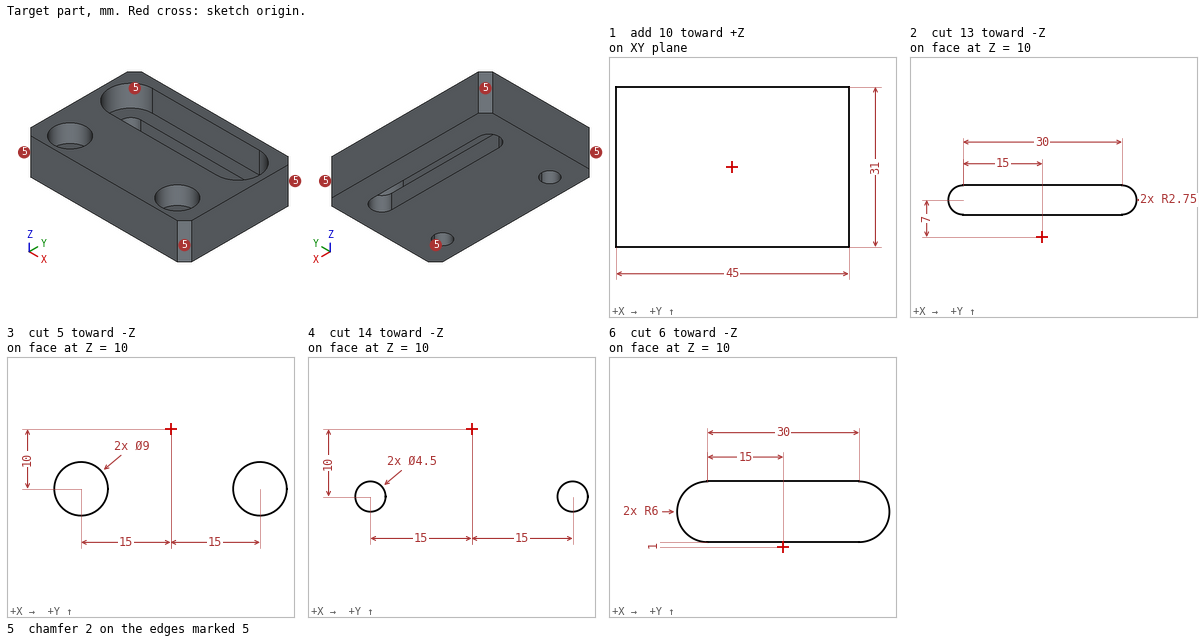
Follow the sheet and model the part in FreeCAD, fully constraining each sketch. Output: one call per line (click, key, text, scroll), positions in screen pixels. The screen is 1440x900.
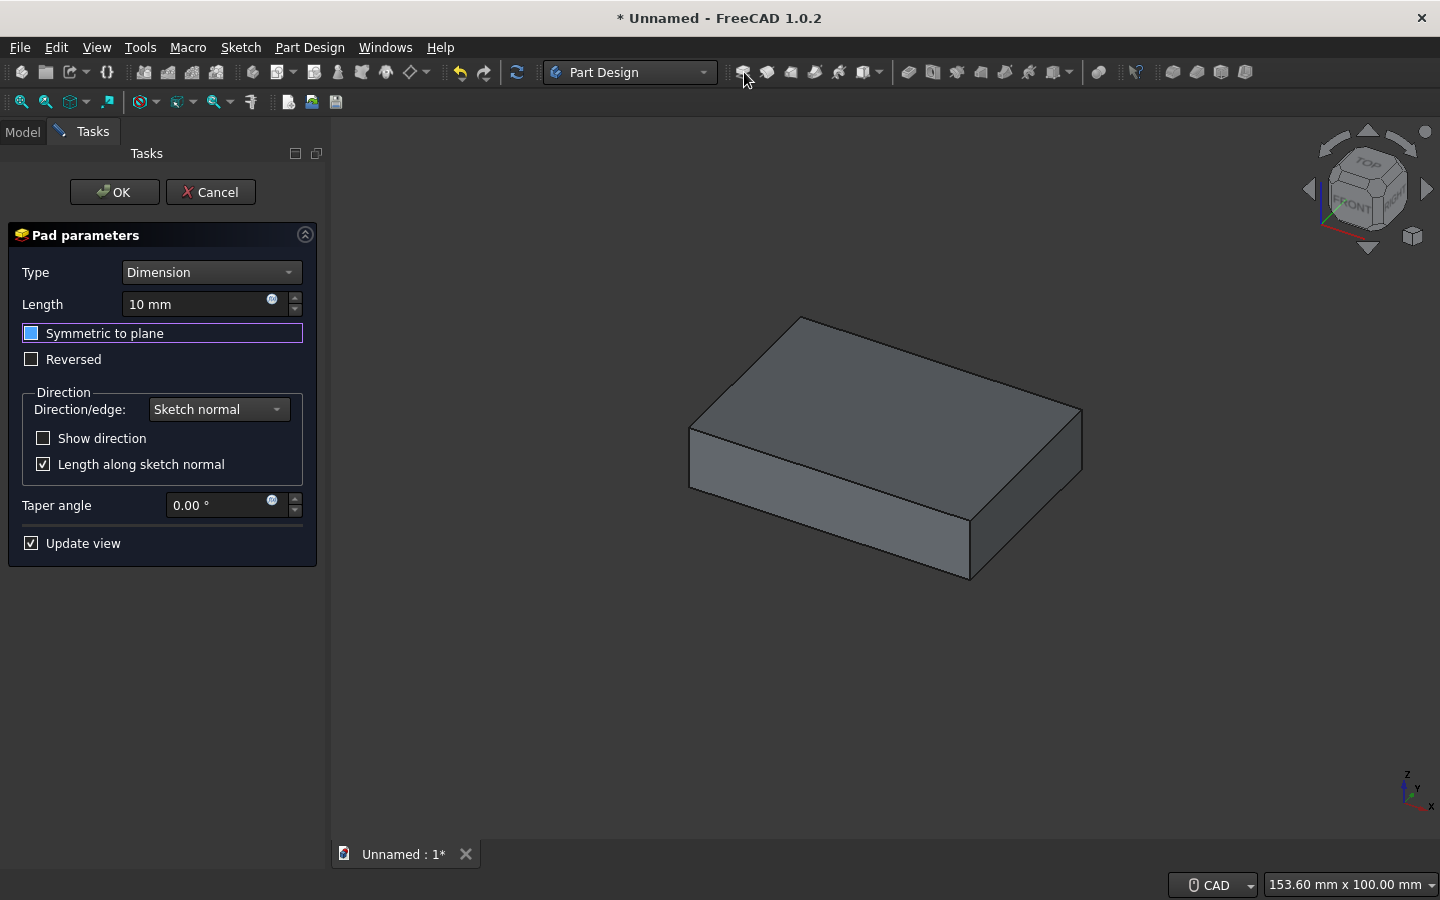
click(115, 192)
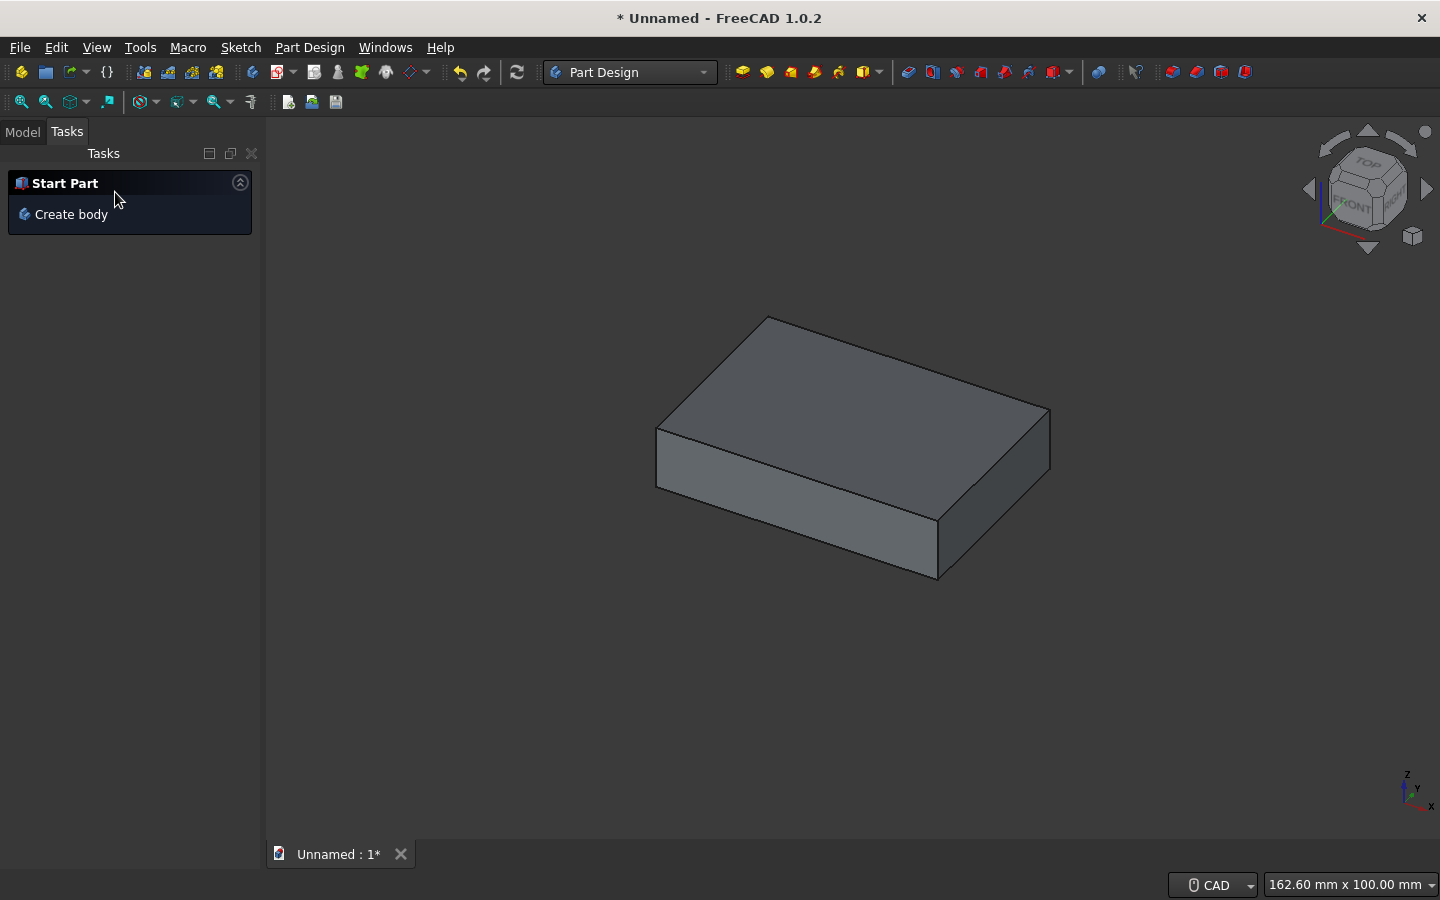
click(22, 102)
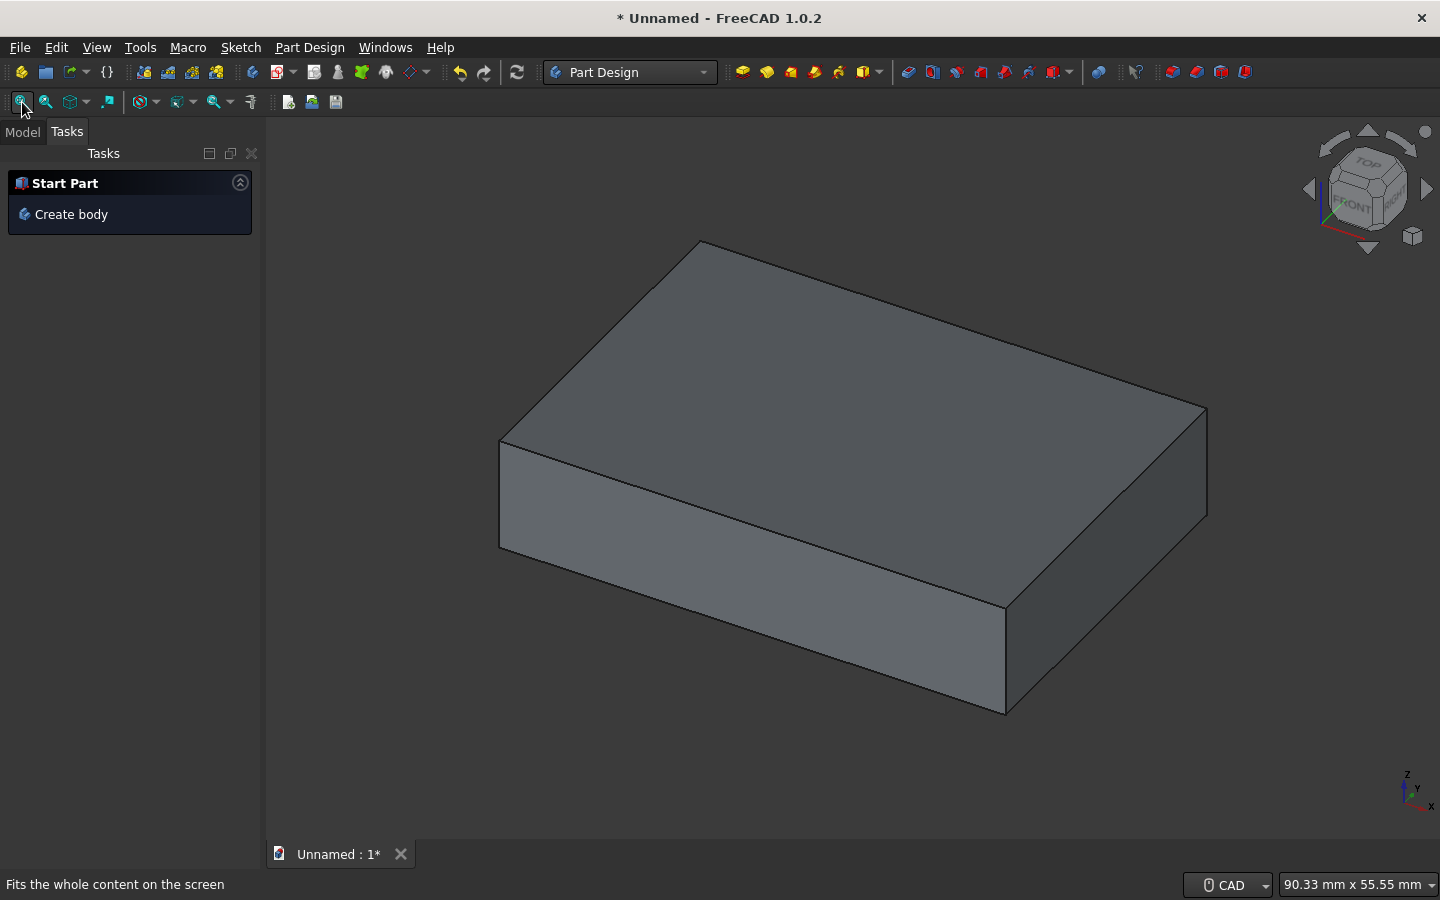
click(925, 448)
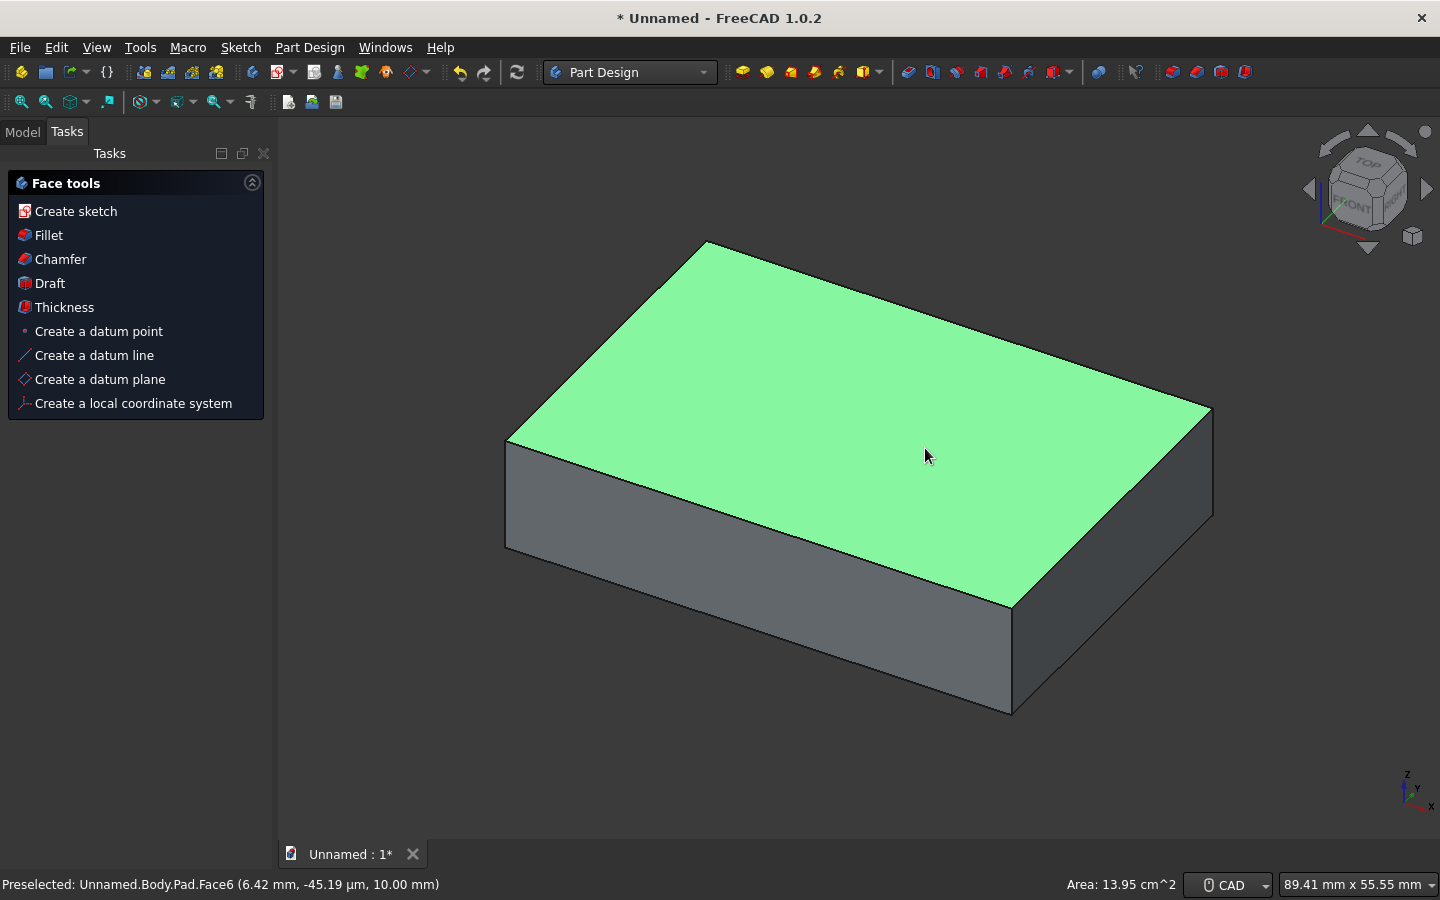
click(278, 72)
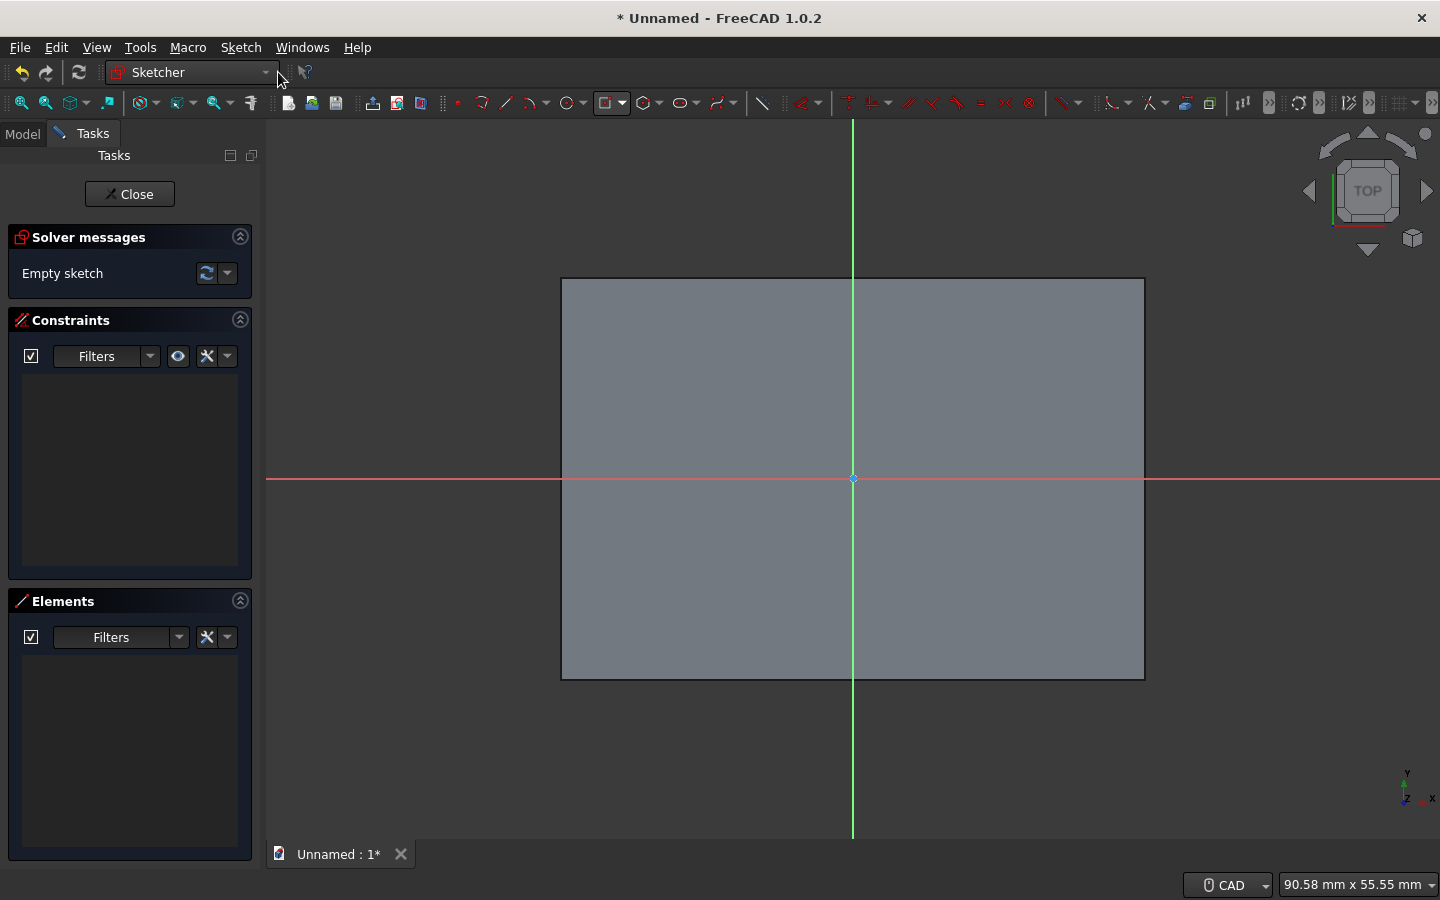
scroll(992, 287, up, 2)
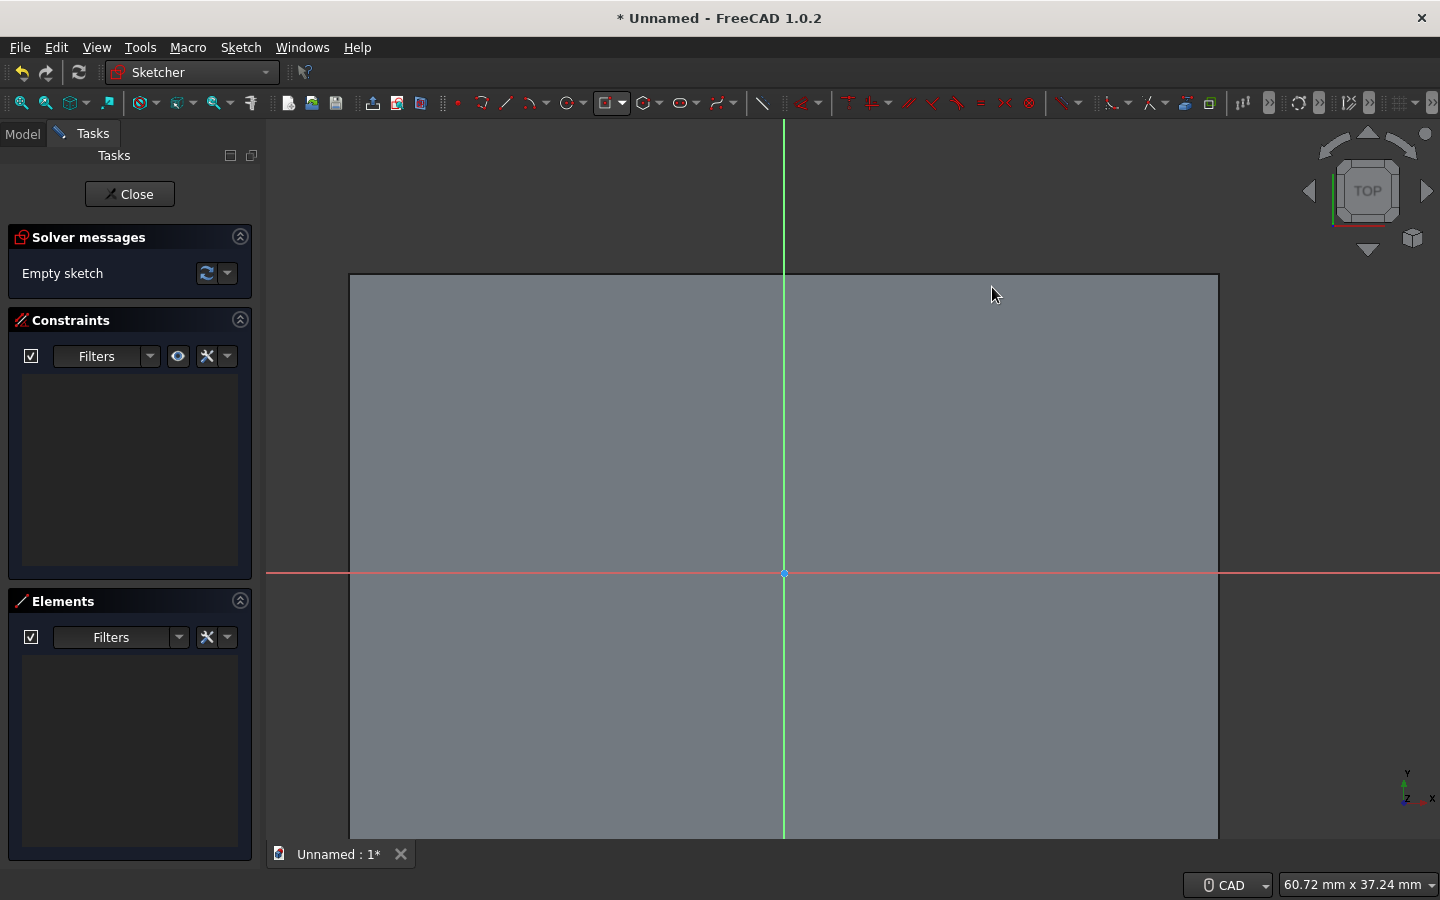
click(680, 104)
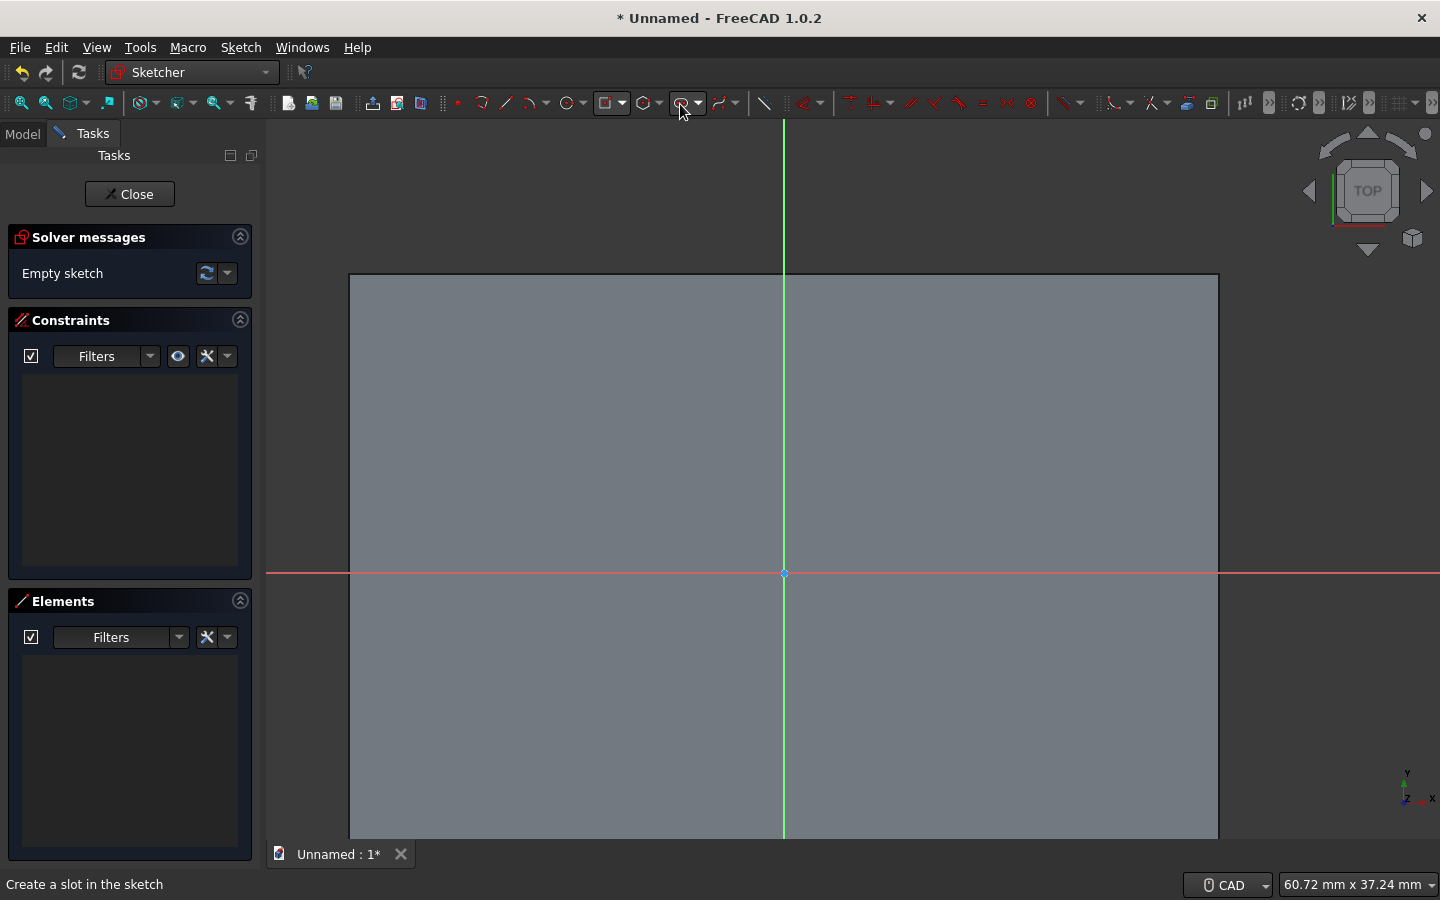
click(494, 438)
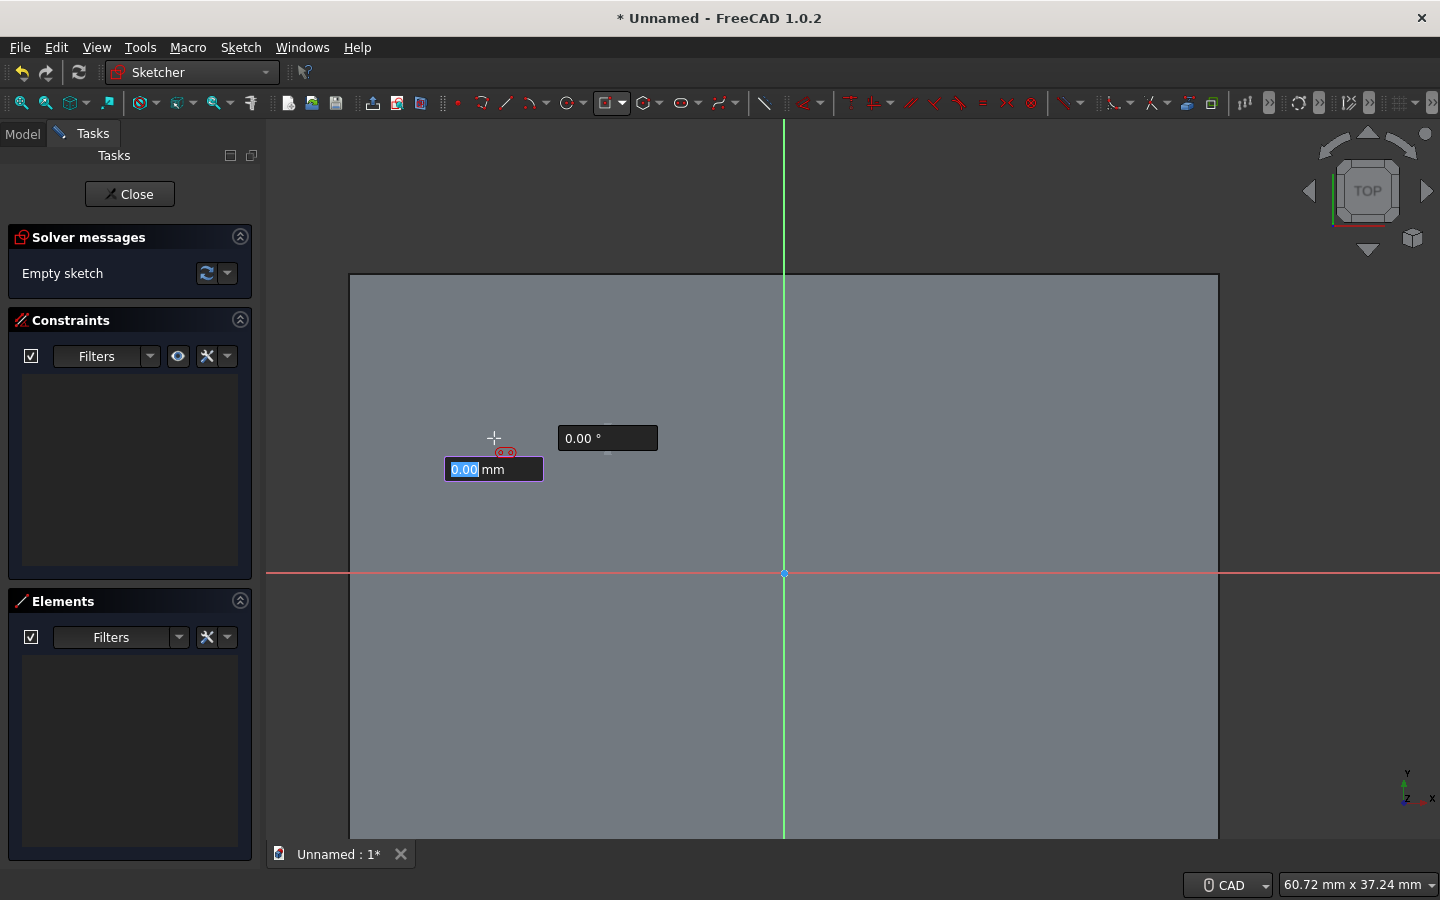
click(1074, 438)